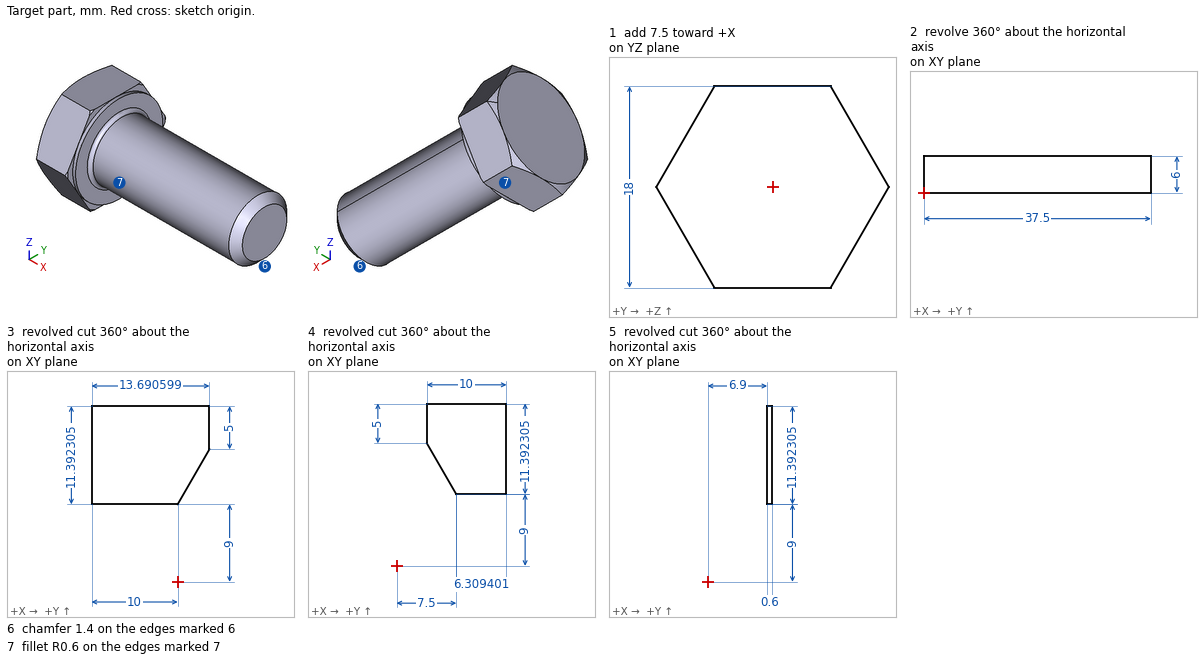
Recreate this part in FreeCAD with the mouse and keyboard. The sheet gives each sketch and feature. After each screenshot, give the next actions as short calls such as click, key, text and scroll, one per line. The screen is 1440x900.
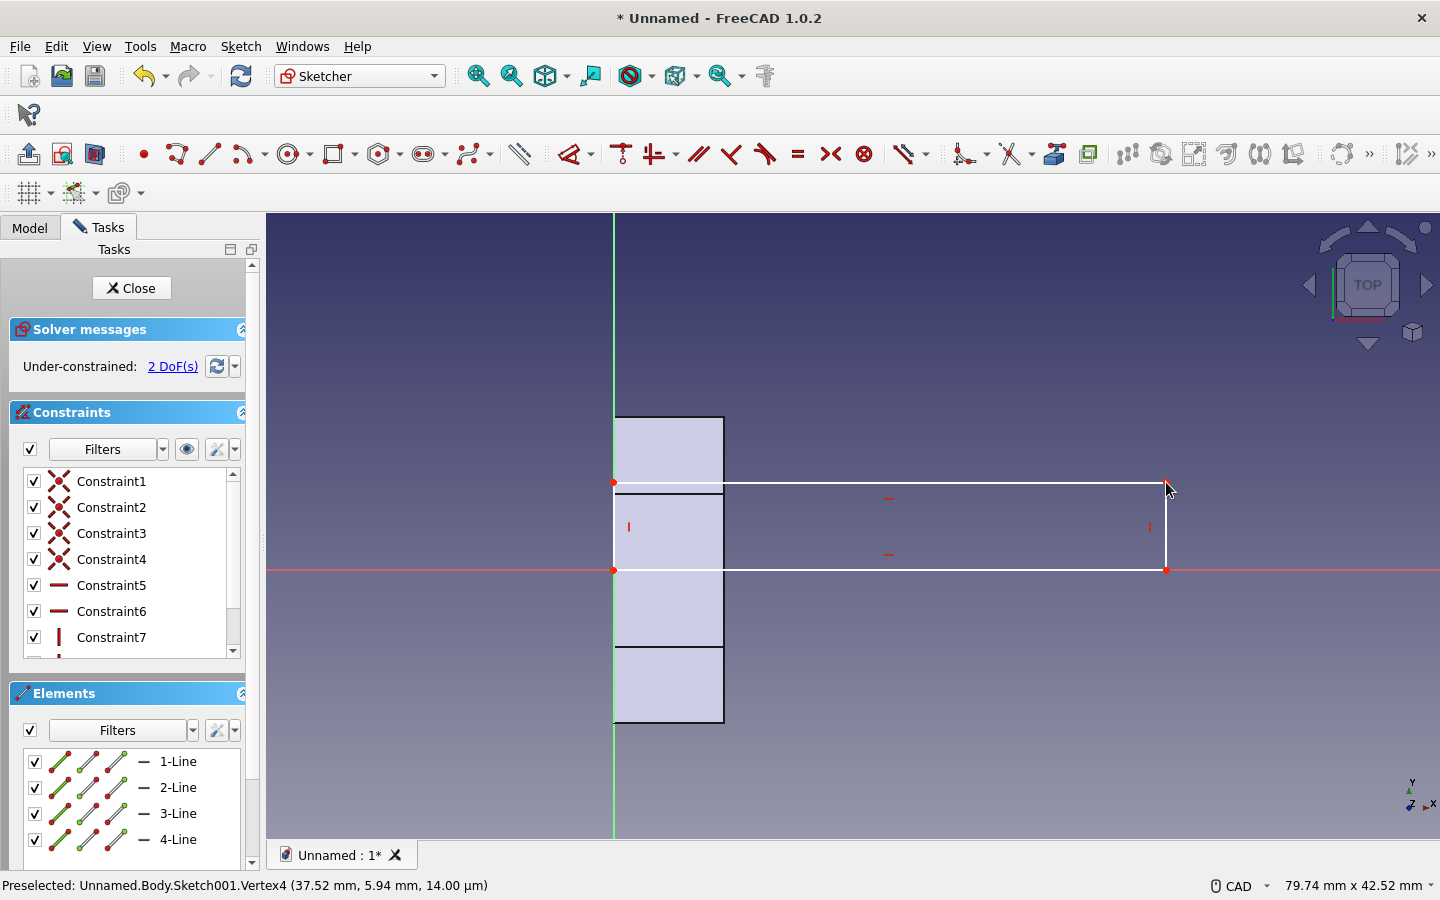
key(d)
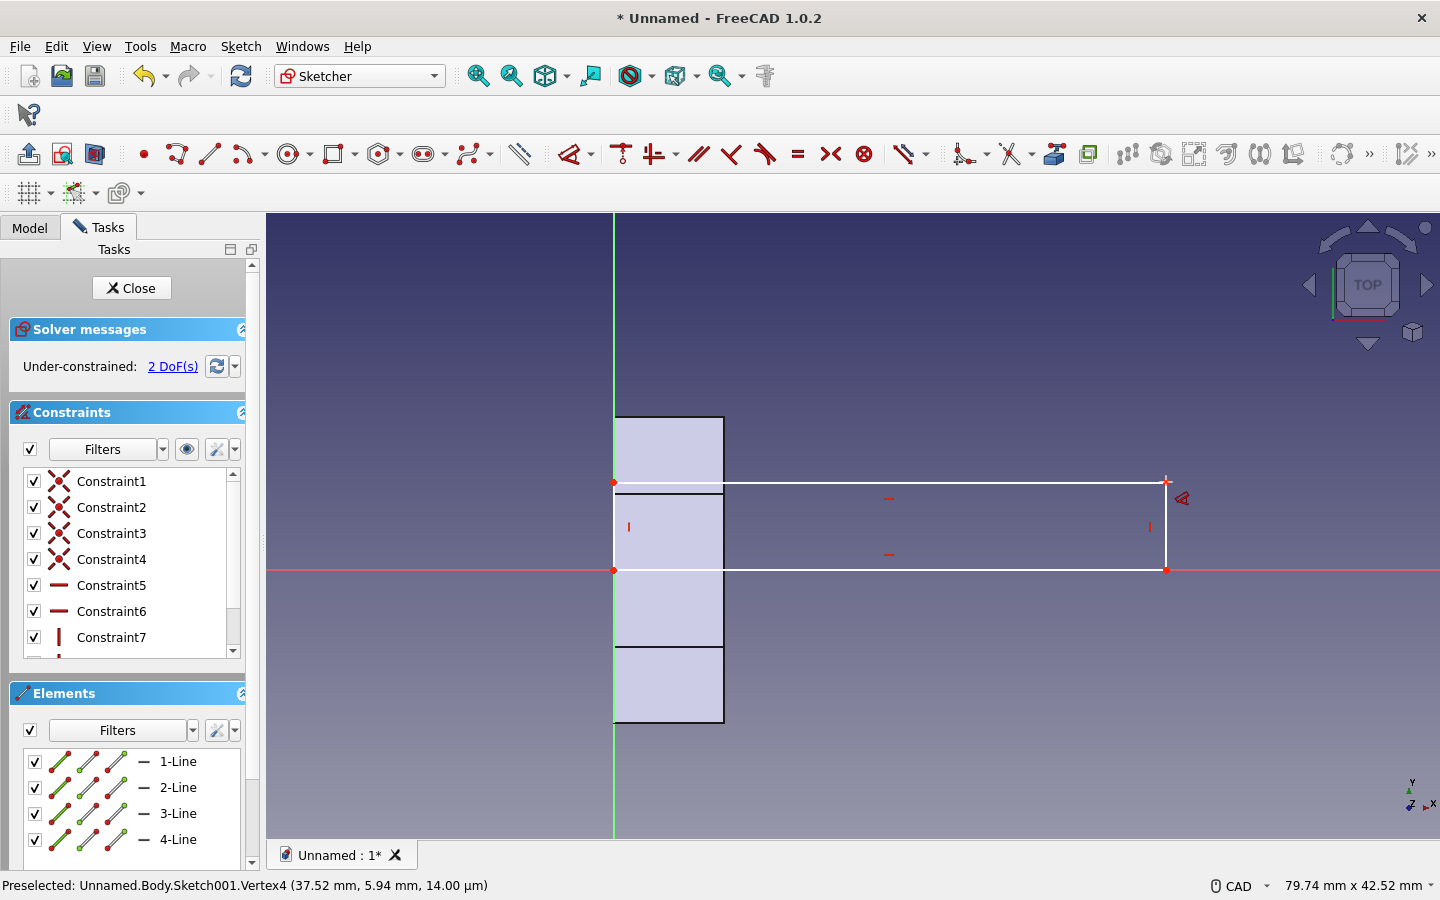
click(1166, 544)
click(1200, 527)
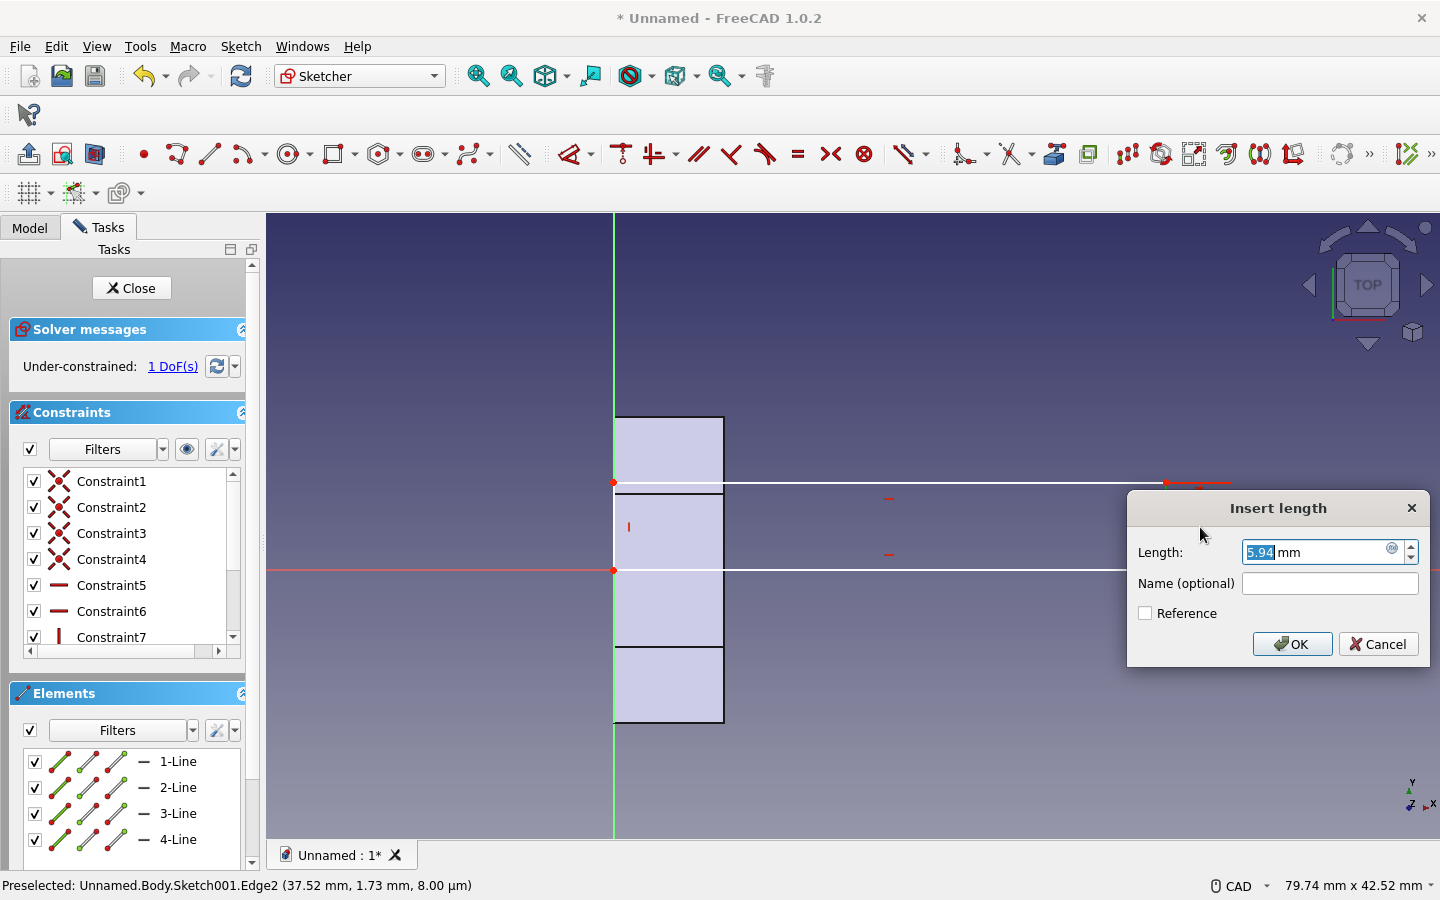
text(6)
key(Return)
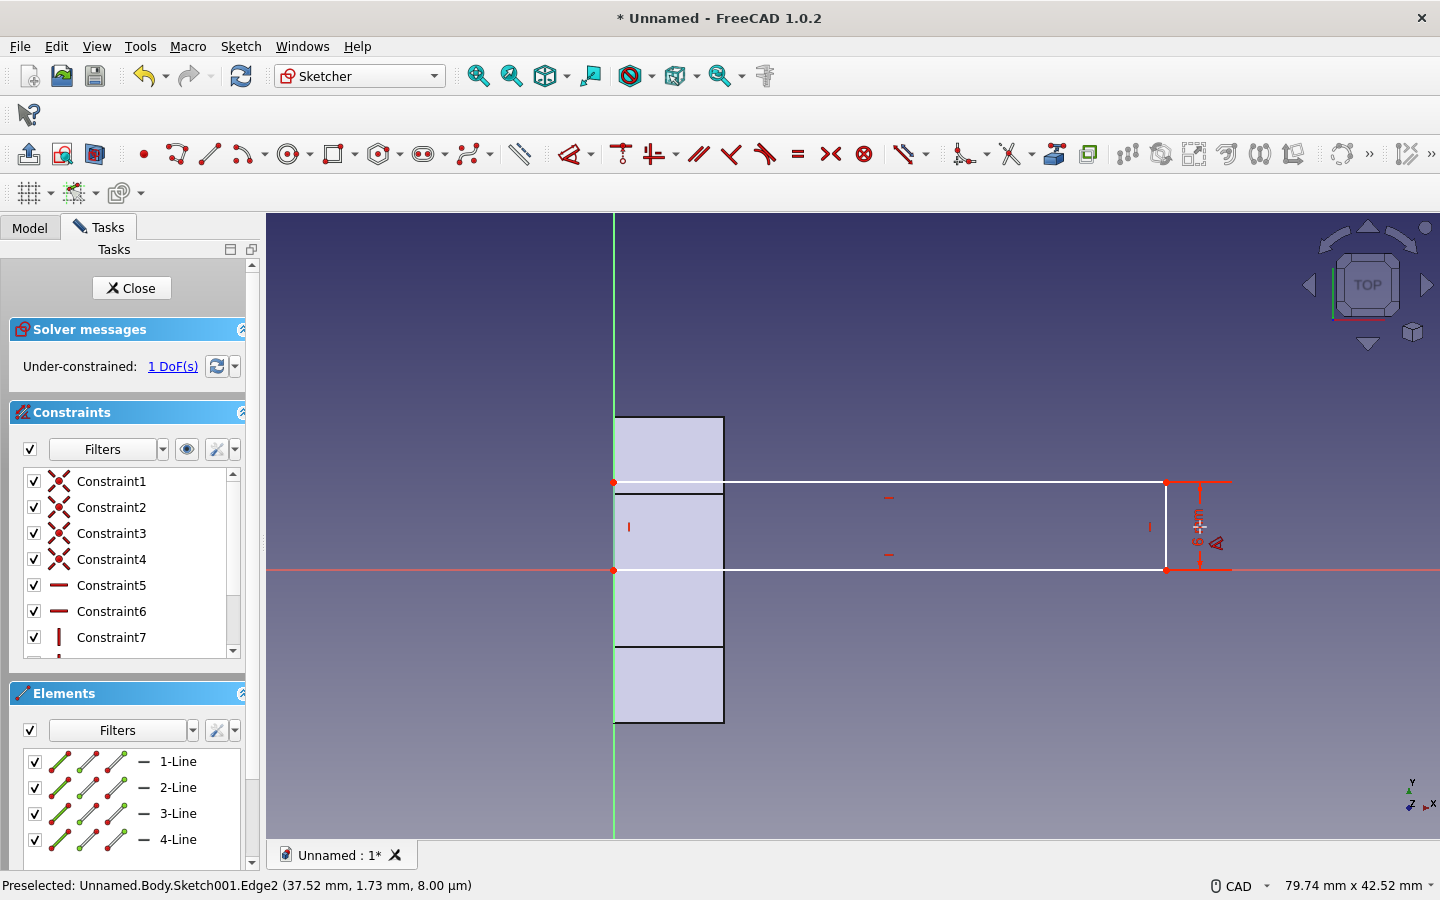
click(779, 570)
click(890, 604)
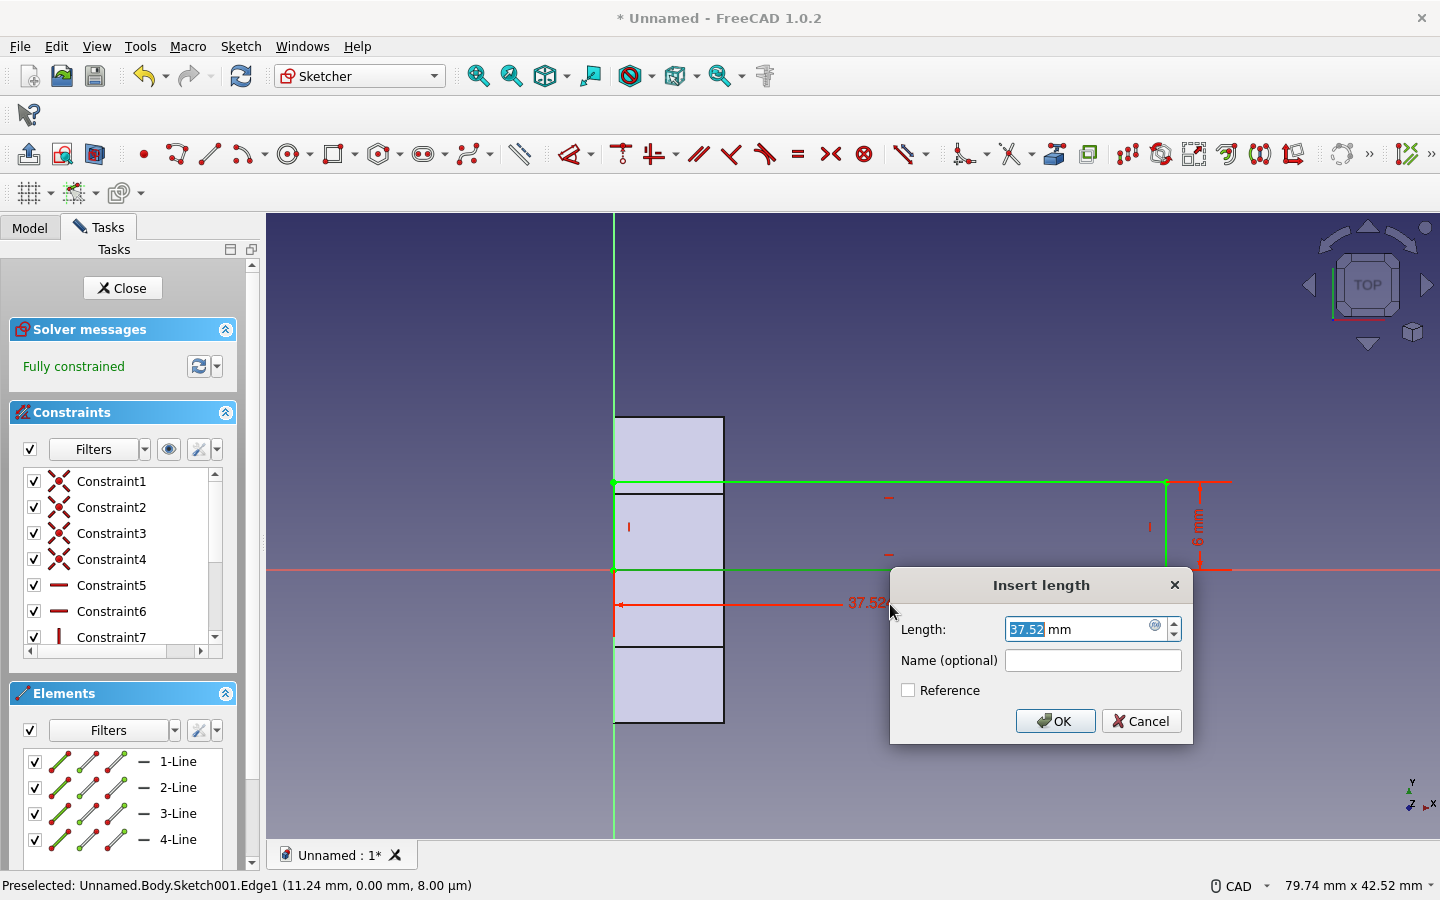
text(37.5)
key(Return)
key(Escape)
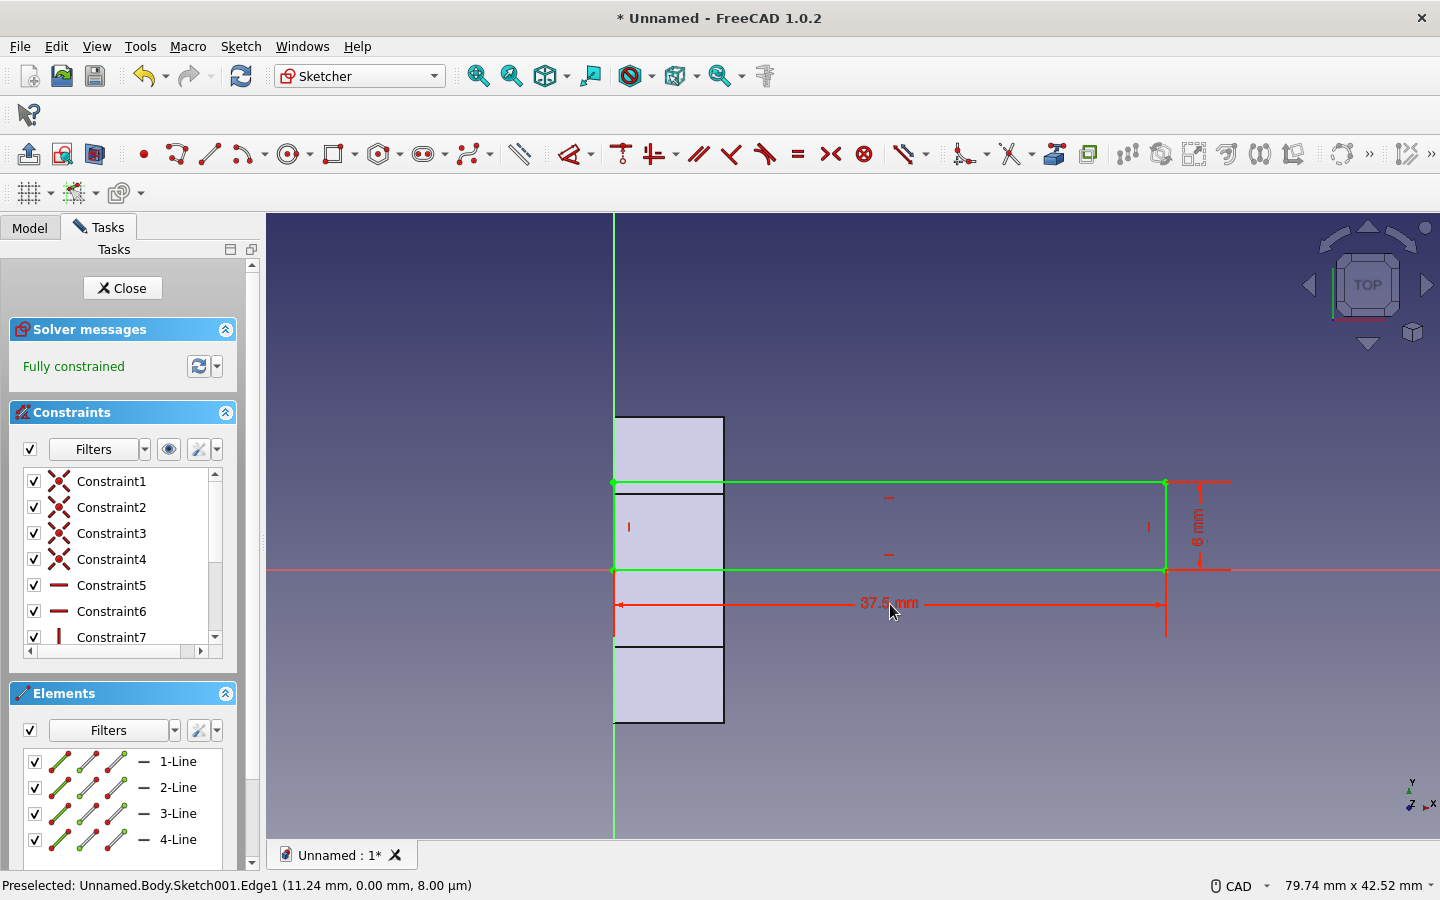
click(123, 288)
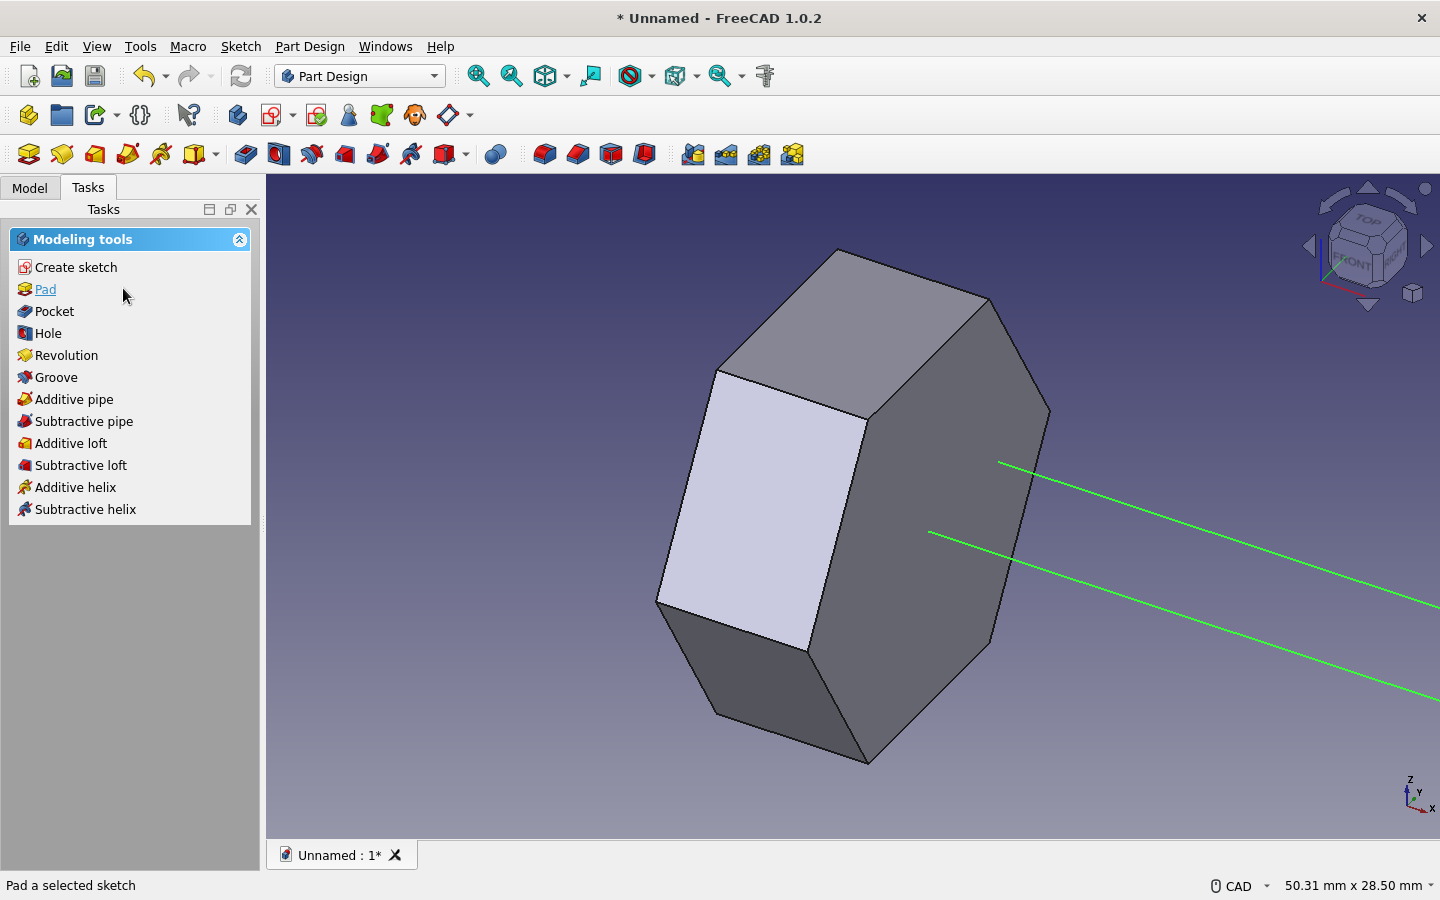
click(62, 154)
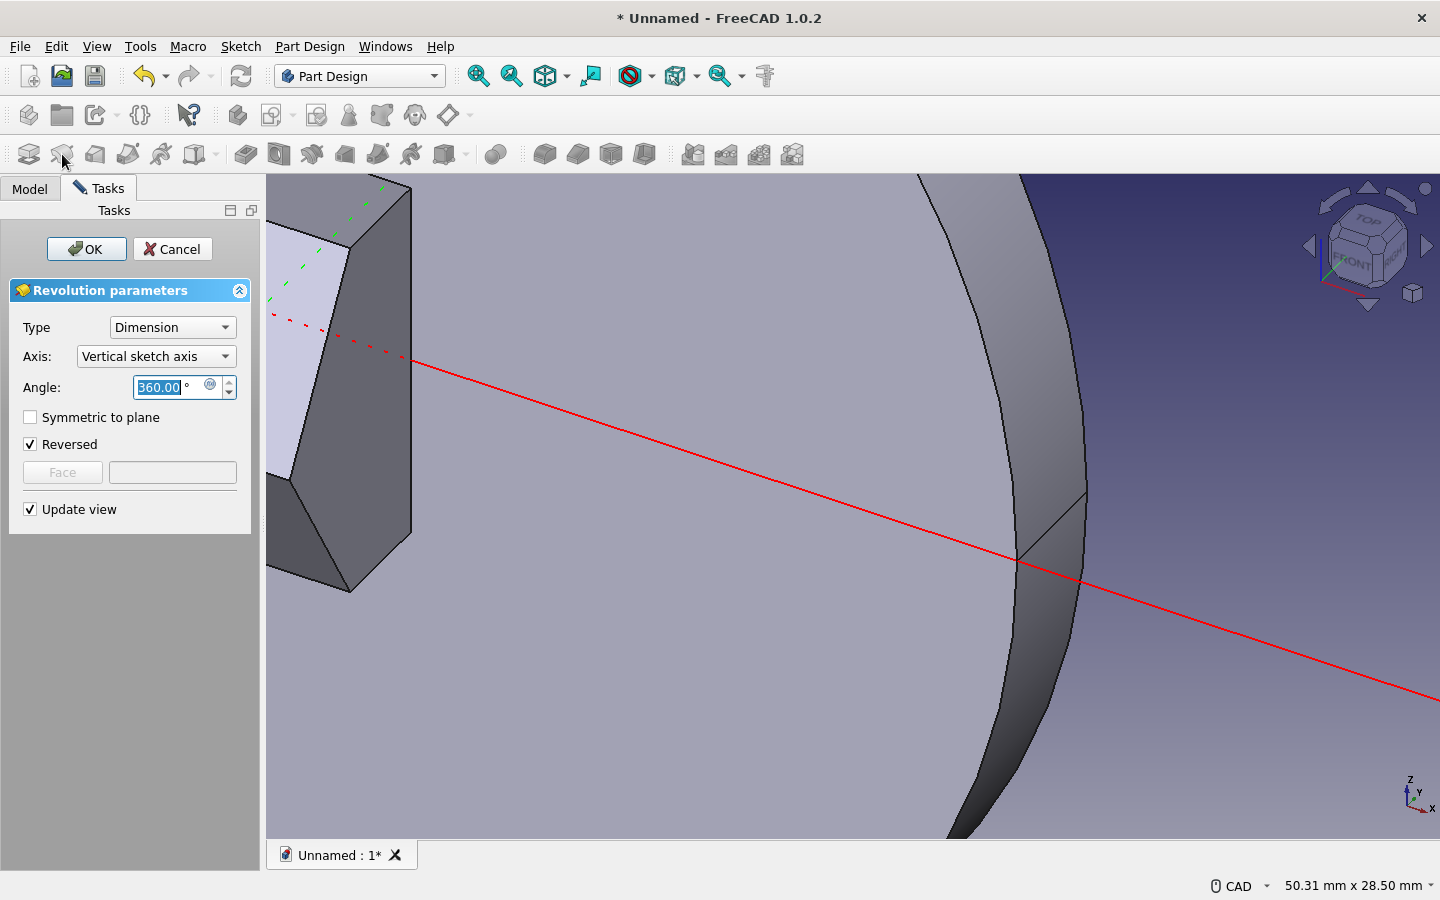
click(157, 356)